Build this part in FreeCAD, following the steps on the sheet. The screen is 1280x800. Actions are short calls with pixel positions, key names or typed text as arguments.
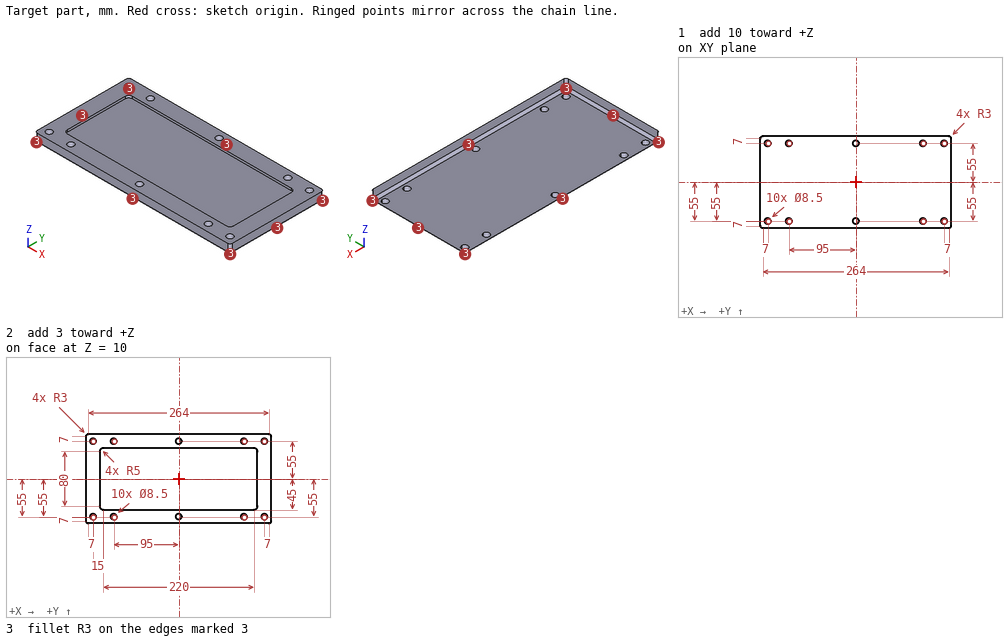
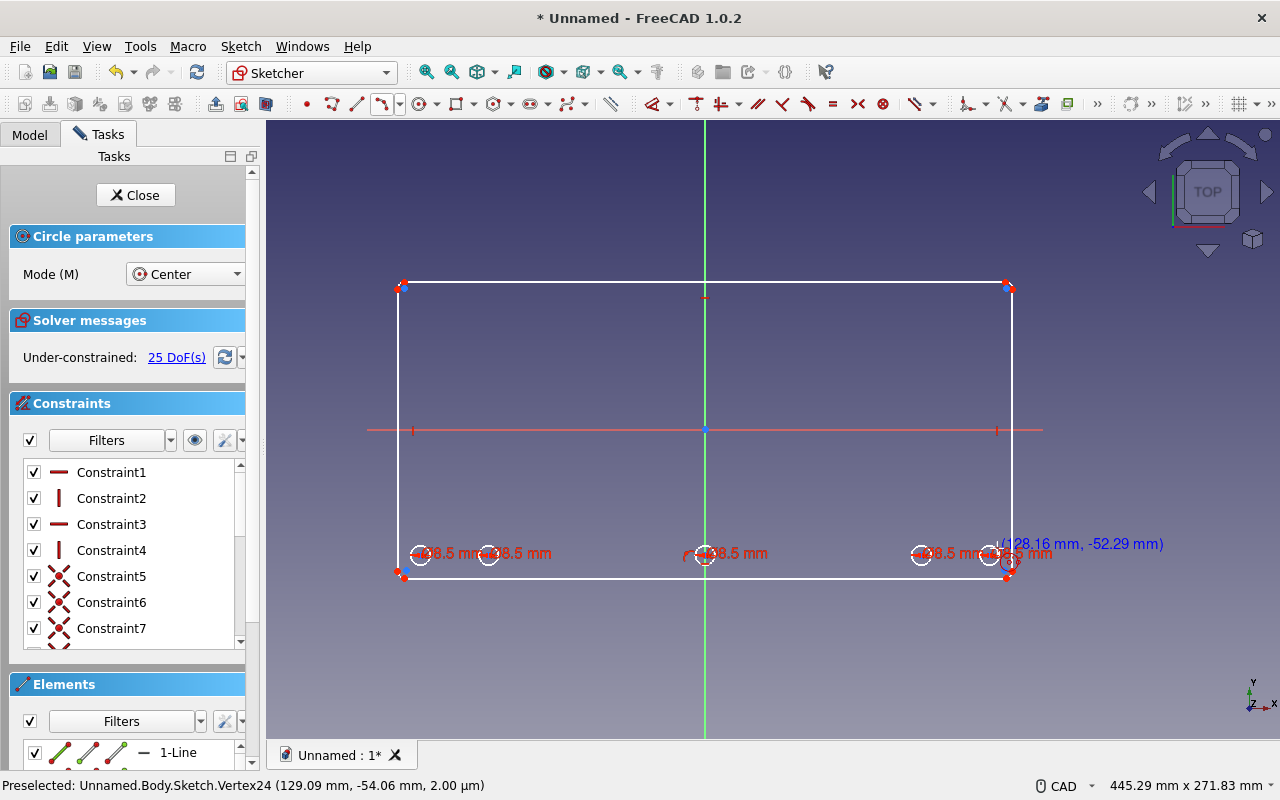
scroll(421, 305, up, 5)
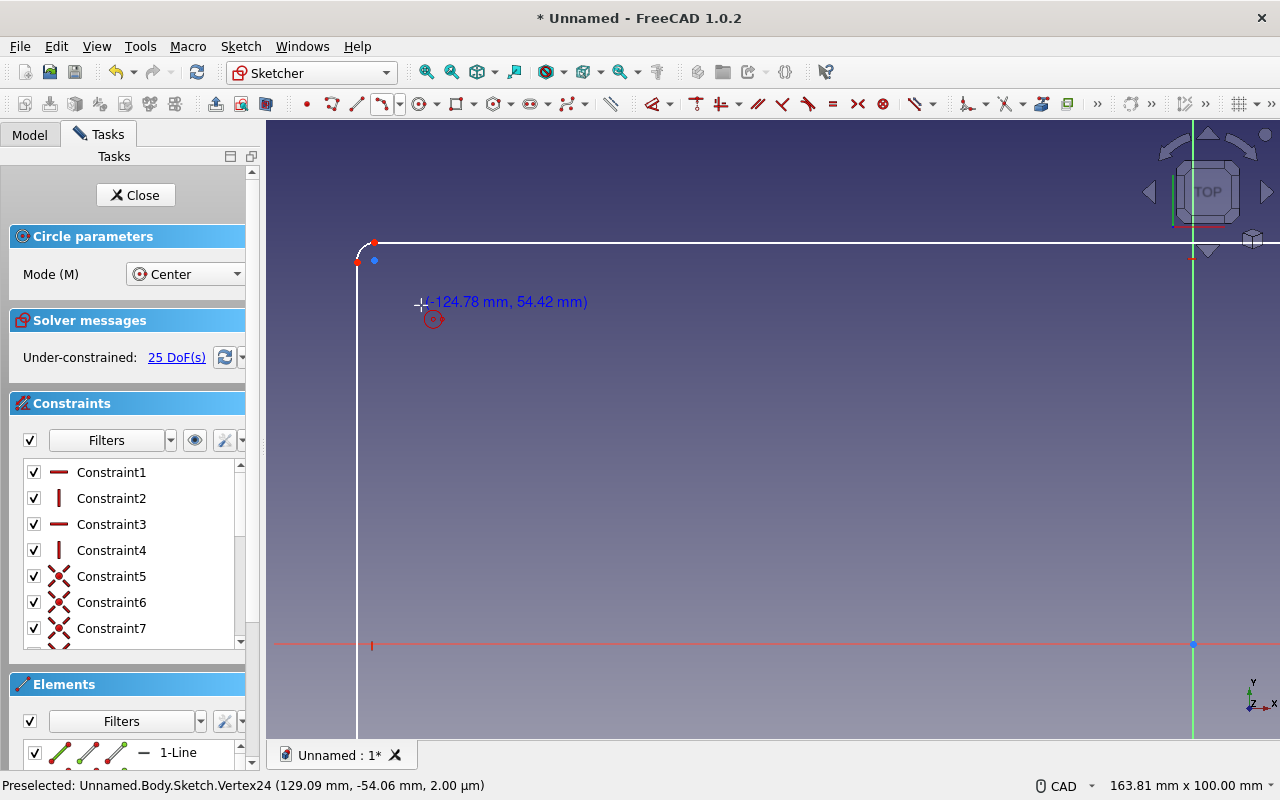
click(419, 304)
move(438, 285)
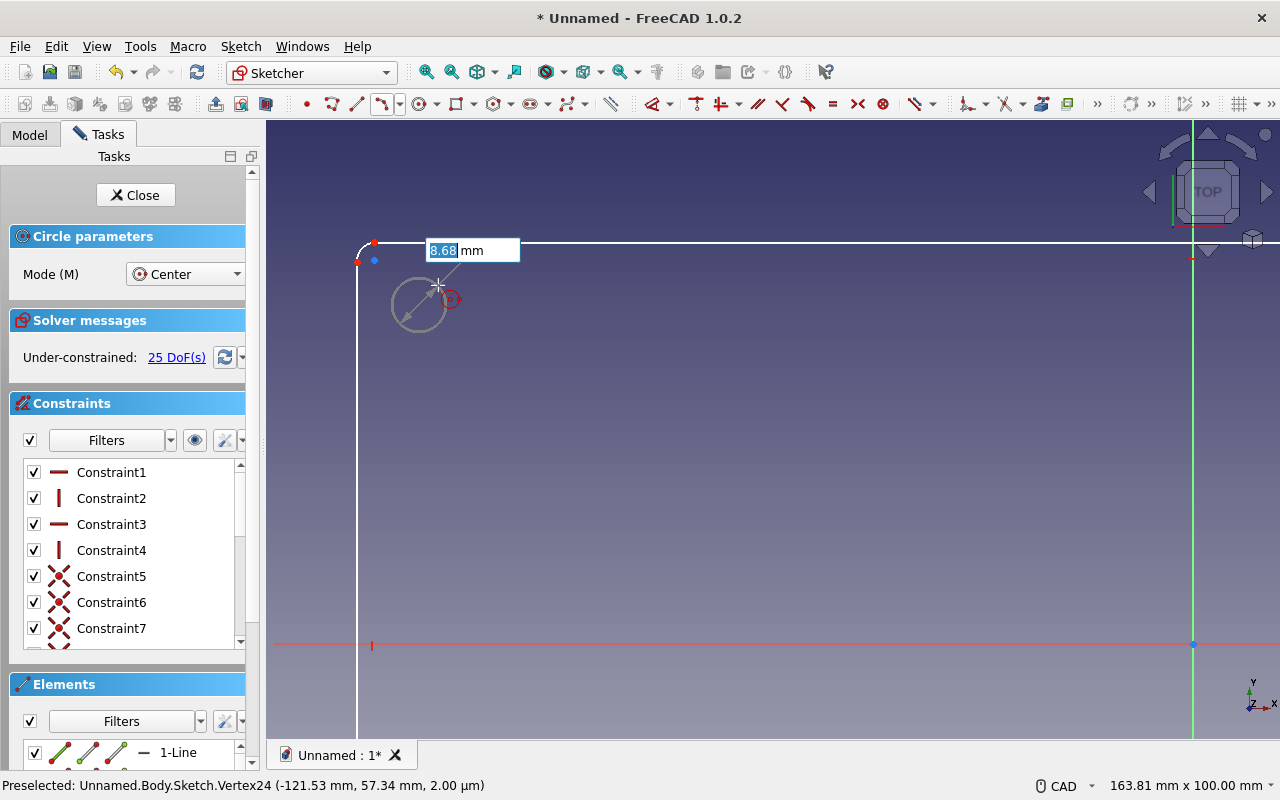
text(8.5)
key(Return)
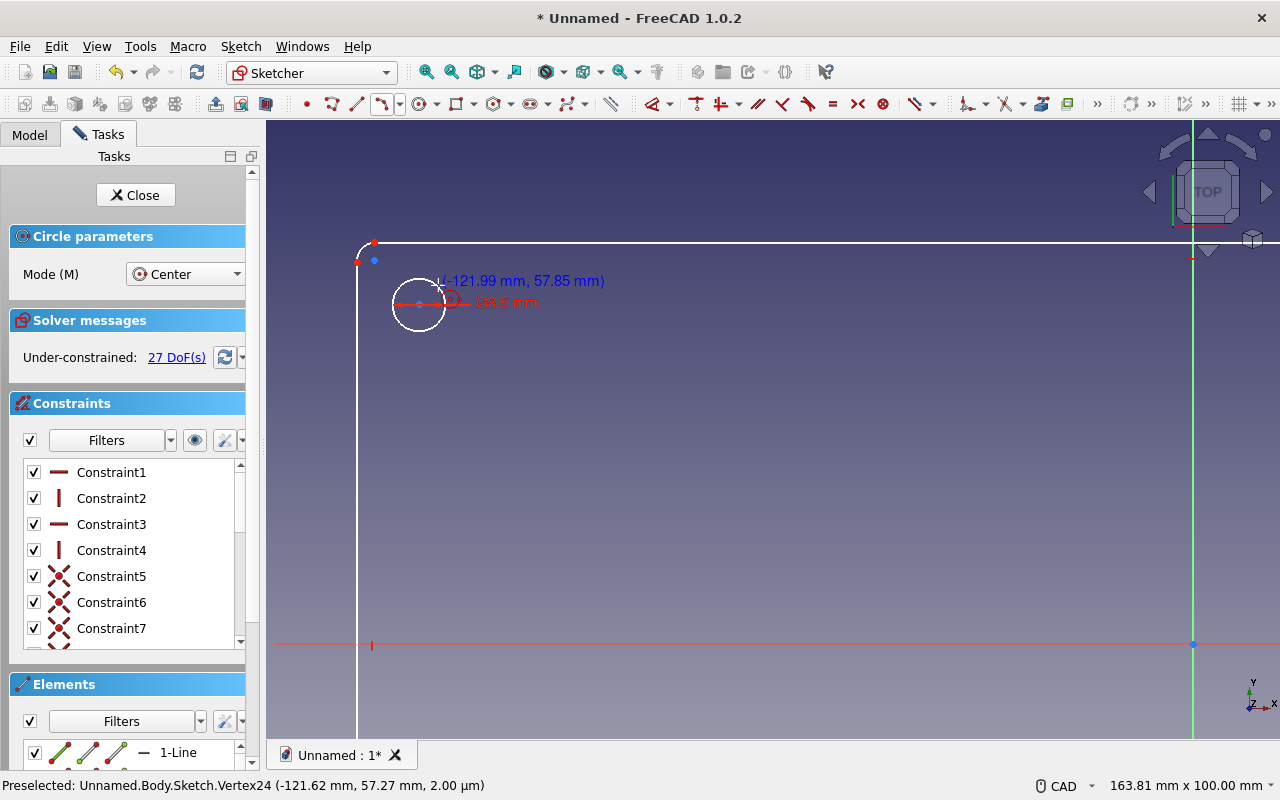
click(605, 304)
move(624, 285)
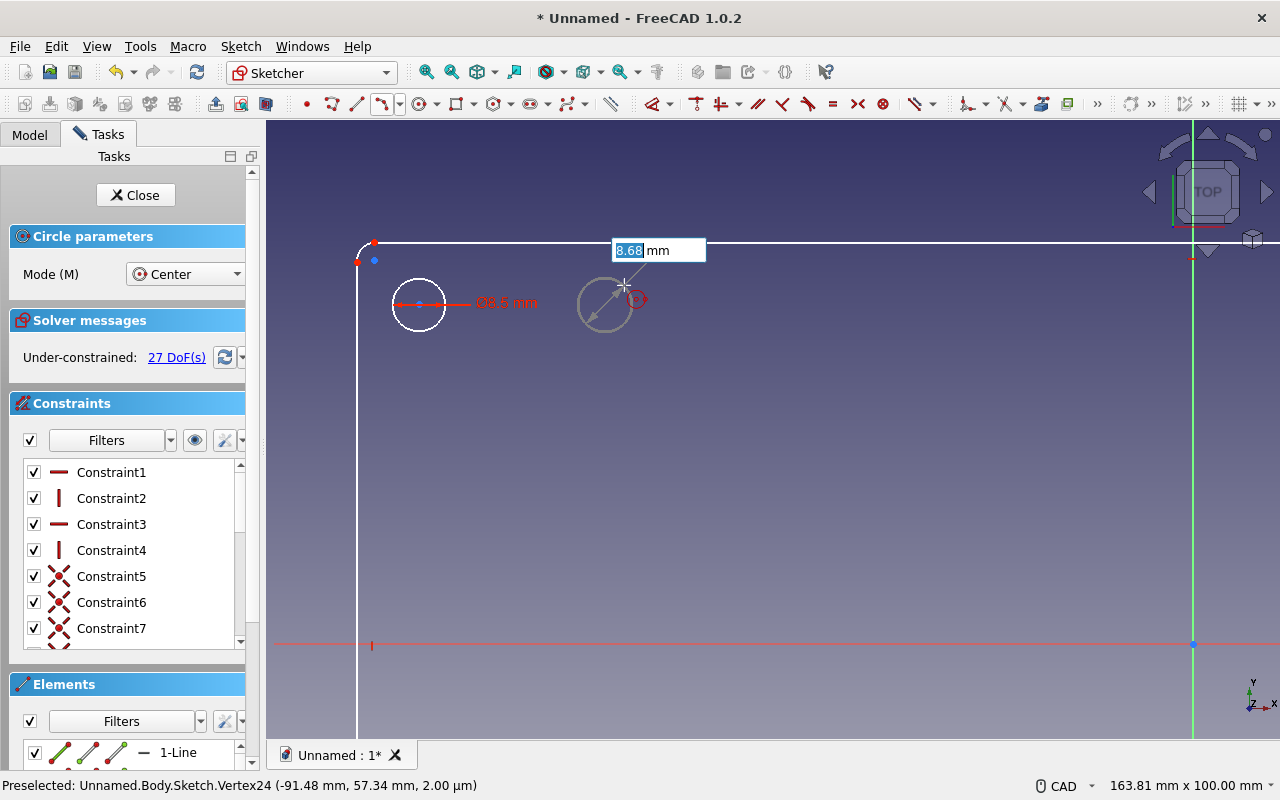
text(8.5)
key(Return)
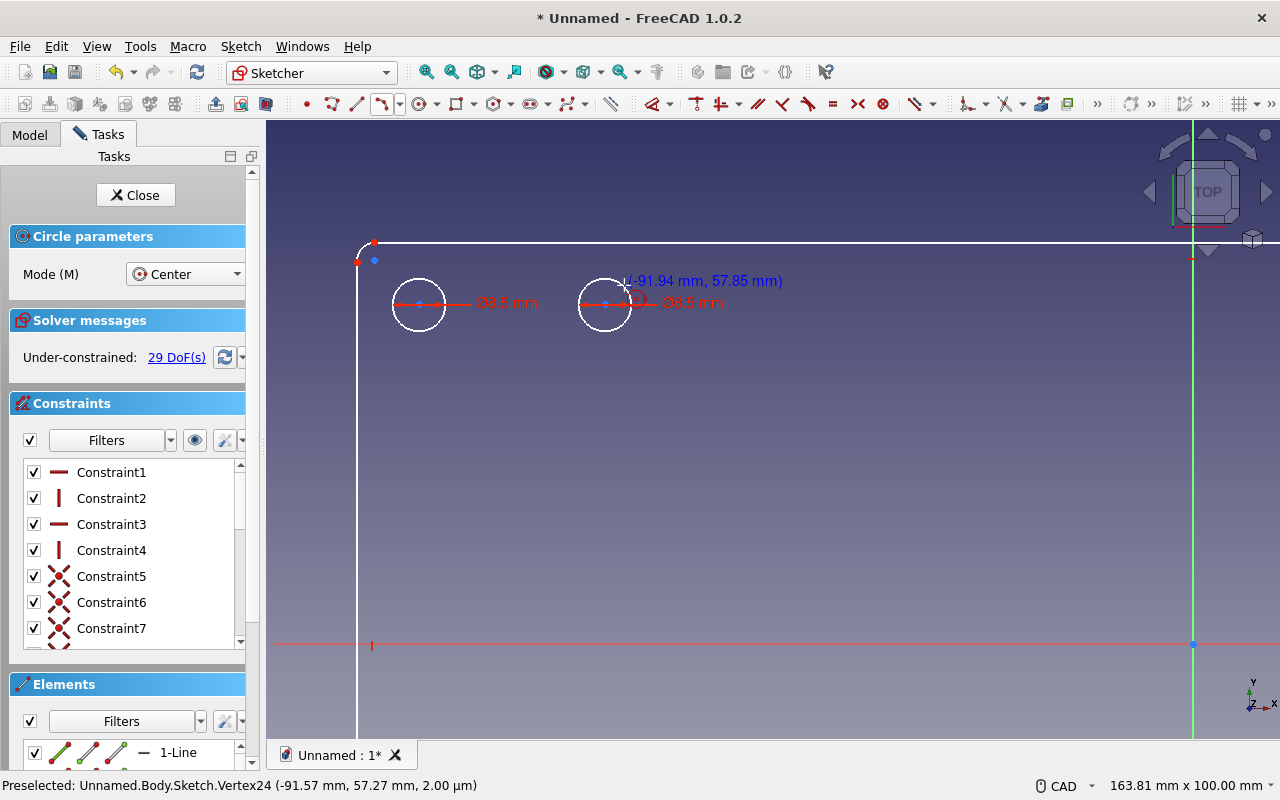
scroll(420, 305, down, 5)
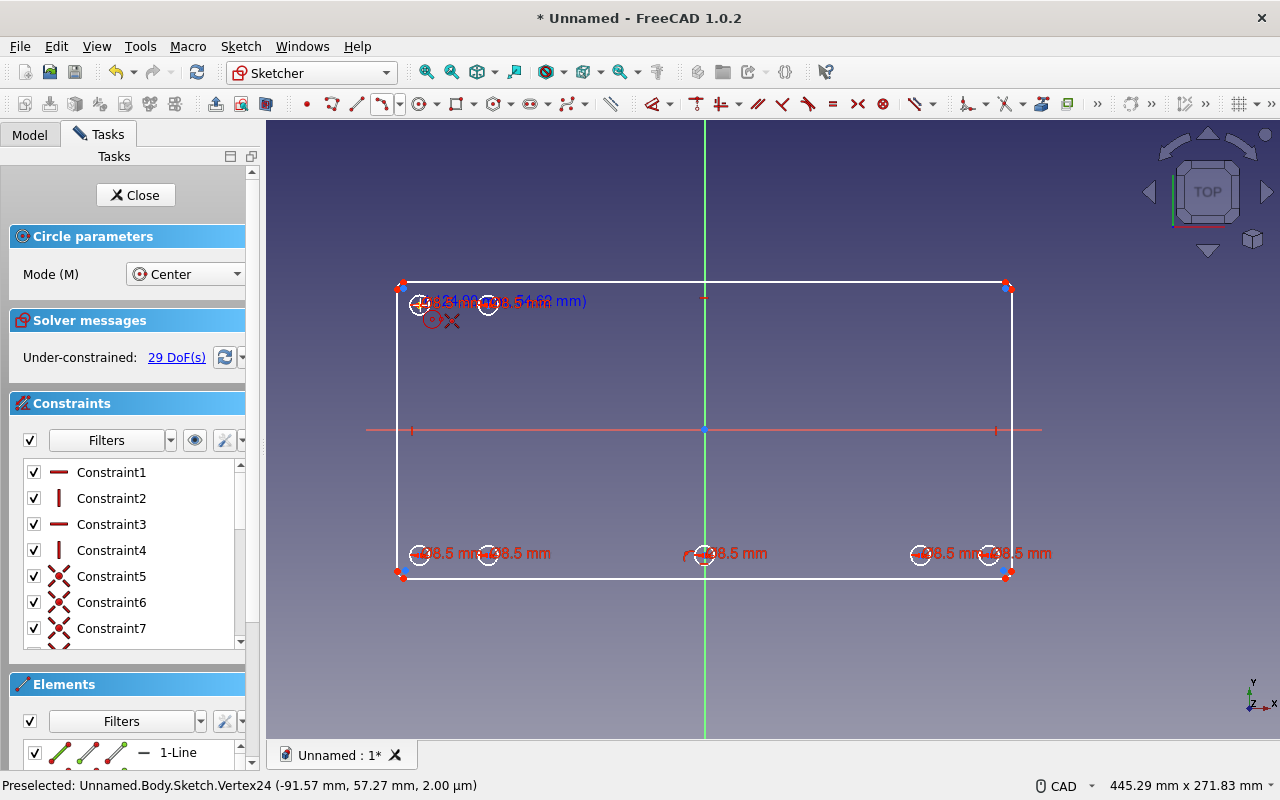
scroll(705, 305, up, 5)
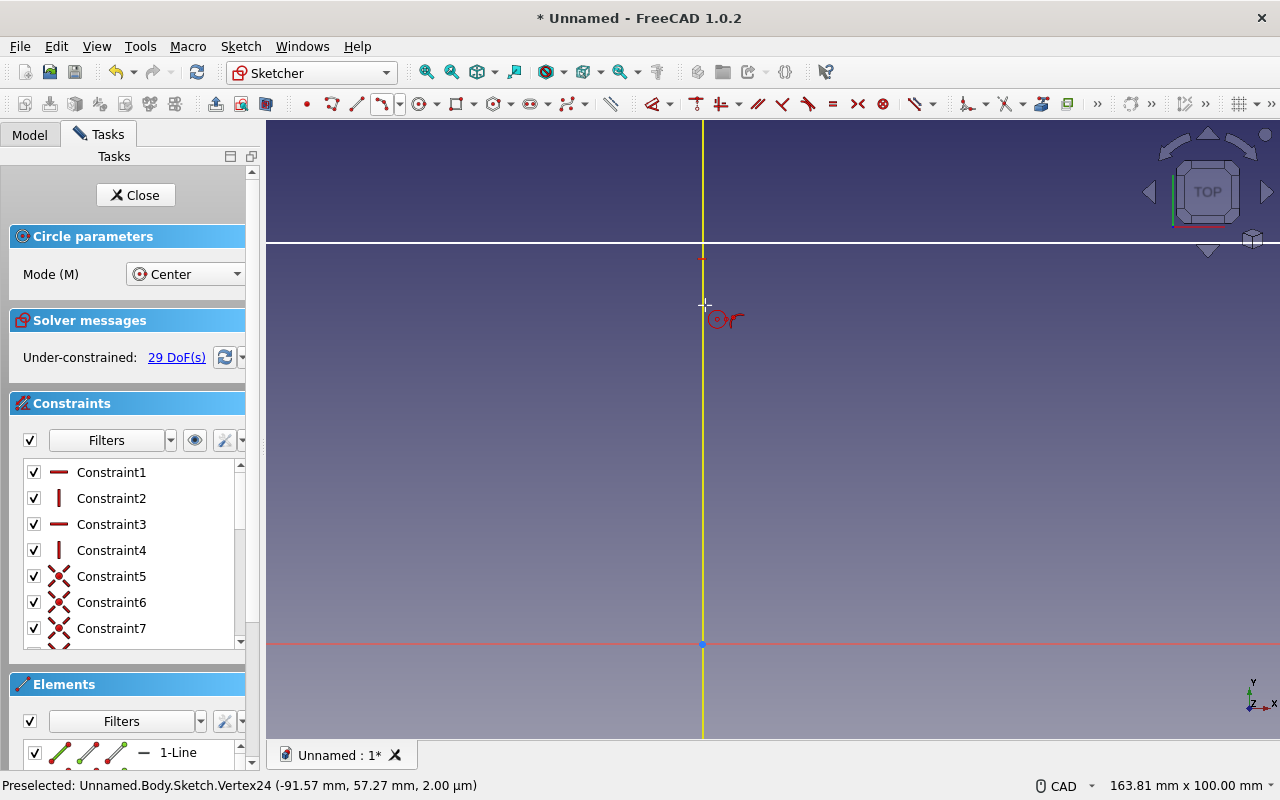
click(703, 304)
move(722, 285)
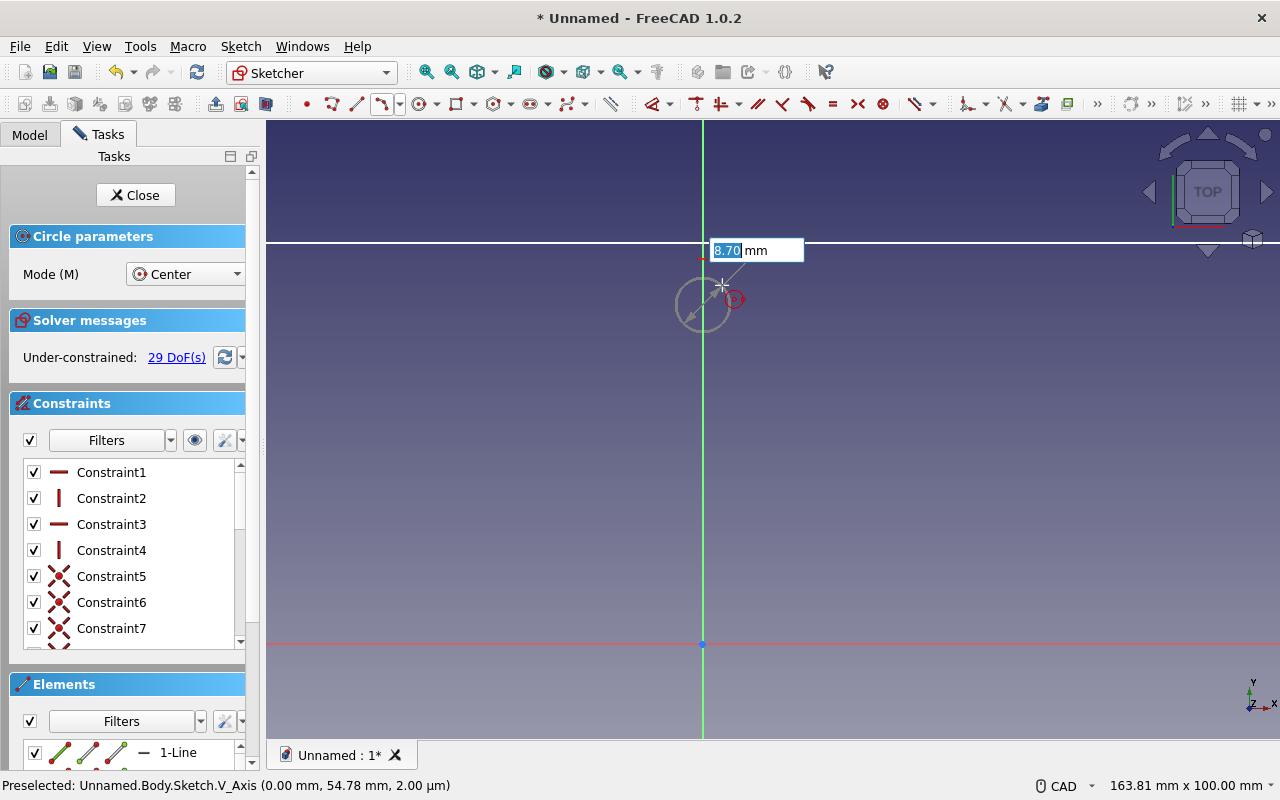
text(8.5)
key(Return)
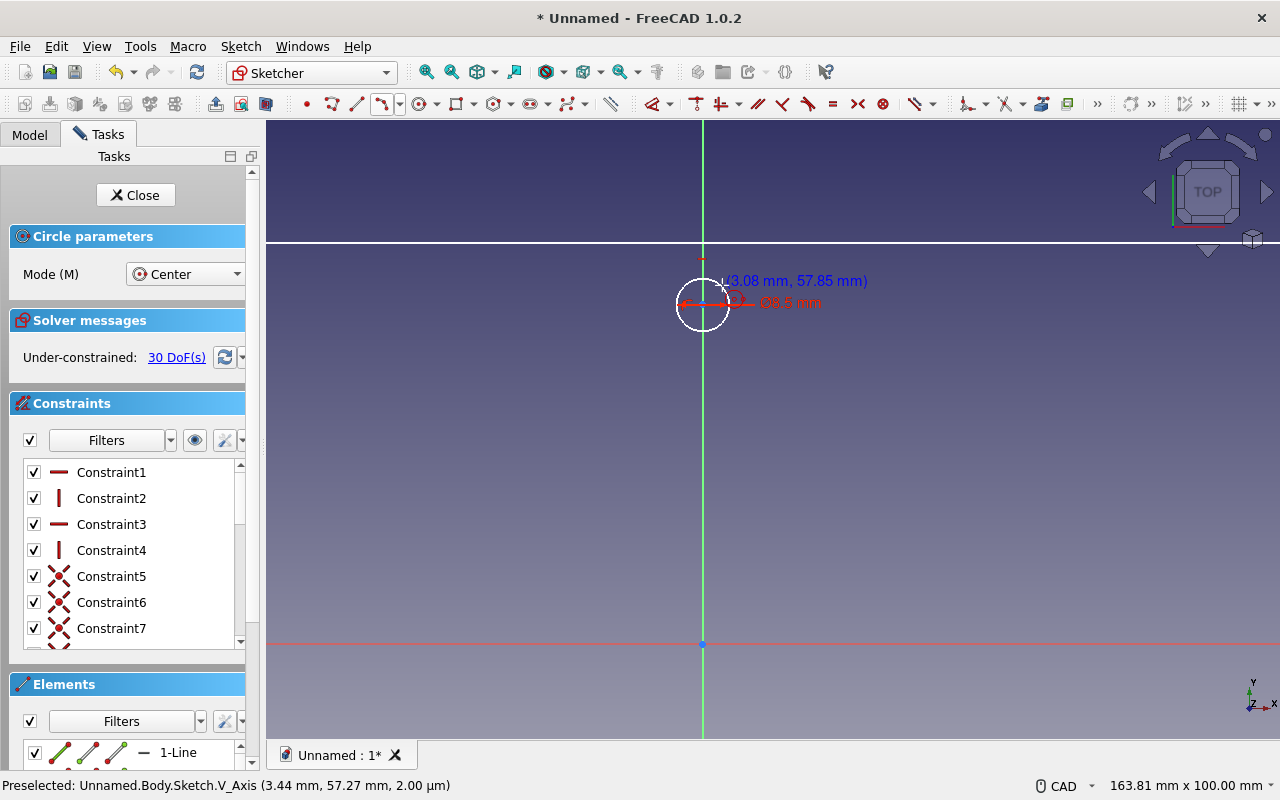
scroll(705, 305, down, 5)